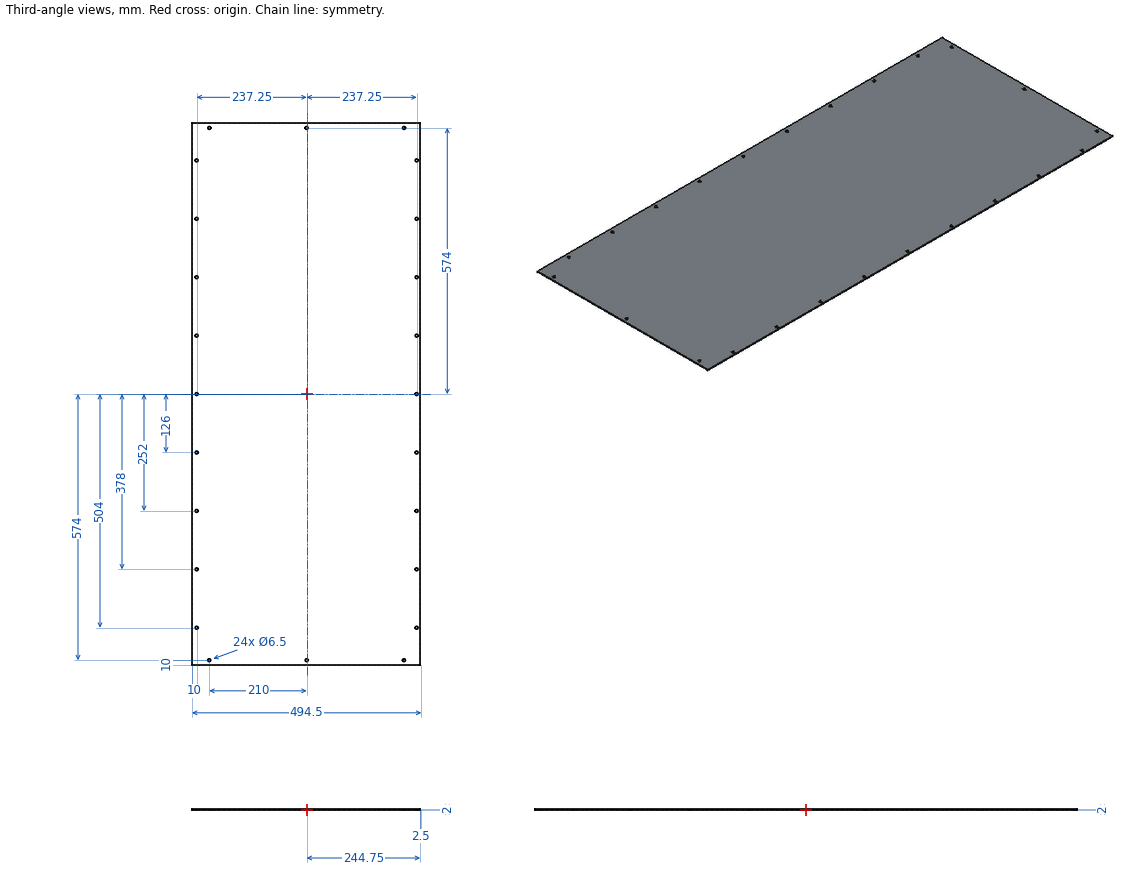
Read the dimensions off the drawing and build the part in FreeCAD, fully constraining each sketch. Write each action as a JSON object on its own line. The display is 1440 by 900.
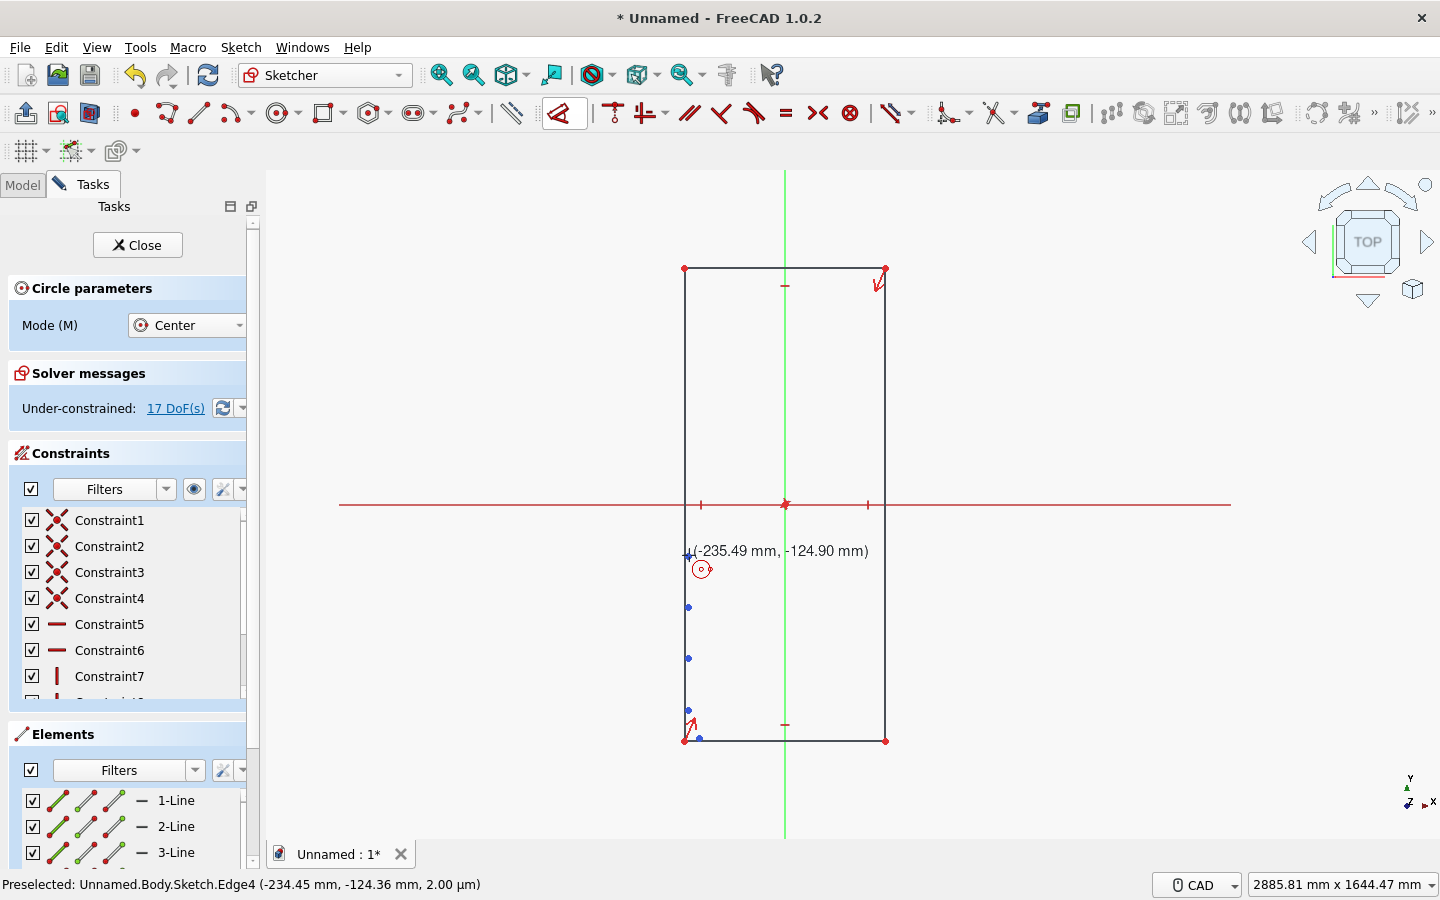
{"action": "scroll", "coordinate": [785, 738], "scroll_direction": "up", "scroll_amount": 15}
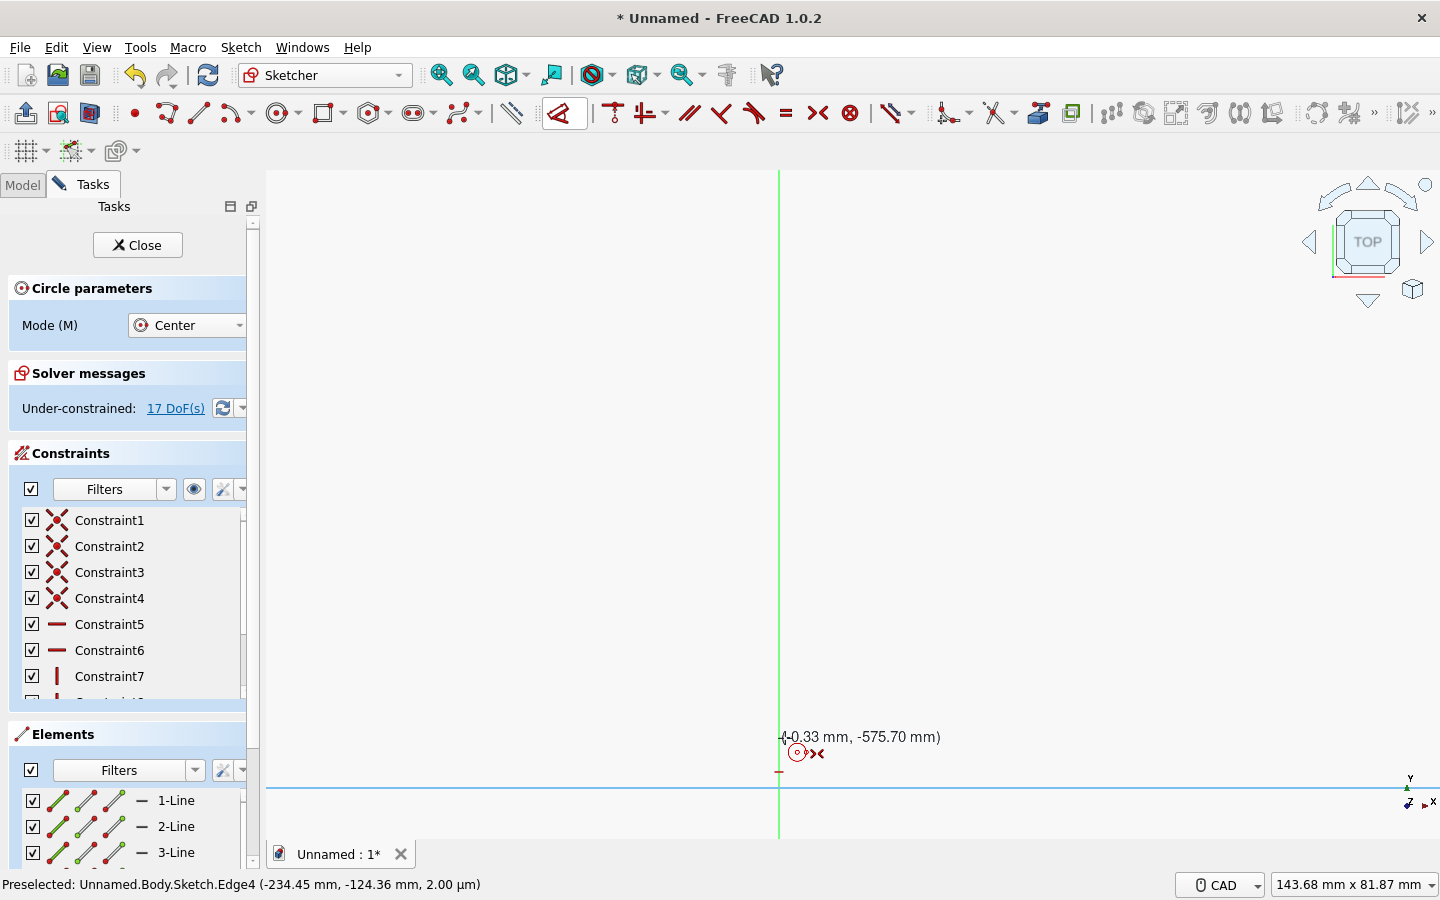
{"action": "scroll", "coordinate": [785, 739], "scroll_direction": "down", "scroll_amount": 15}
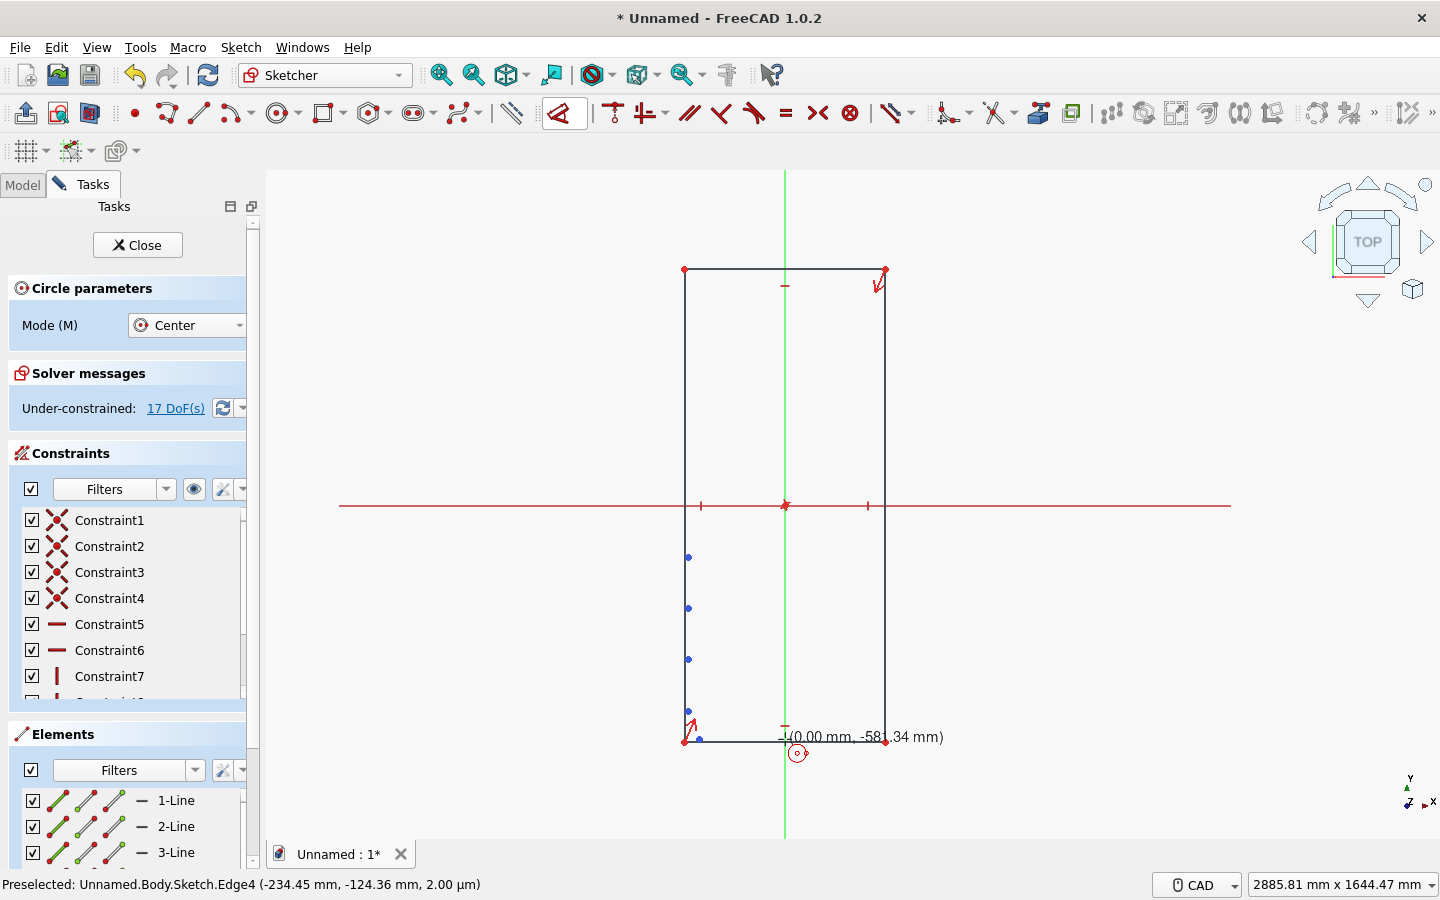
{"action": "scroll", "coordinate": [785, 739], "scroll_direction": "up", "scroll_amount": 7}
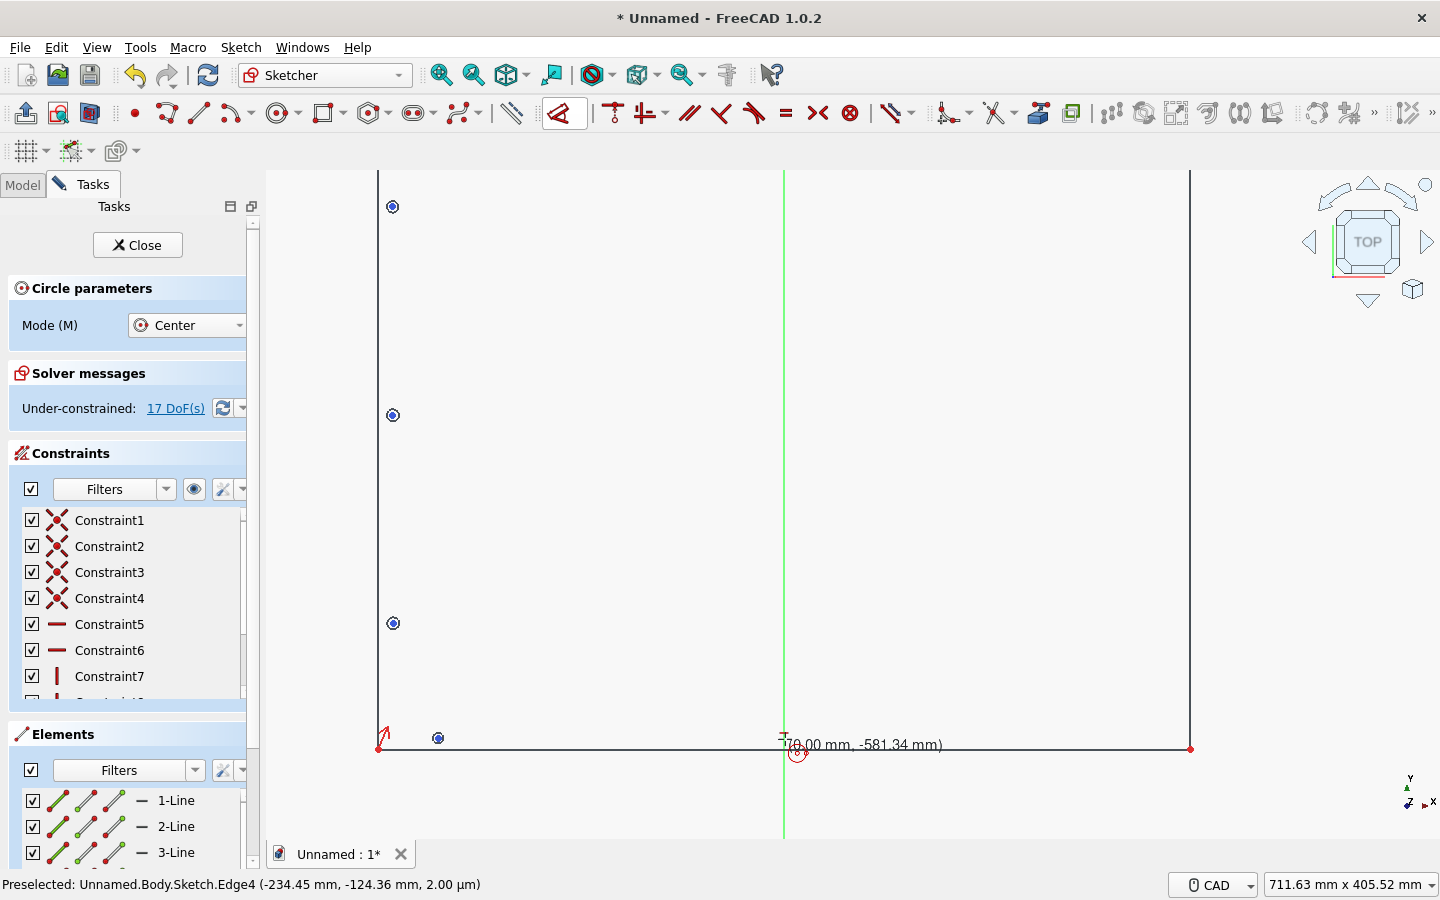
{"action": "left_click", "coordinate": [784, 737]}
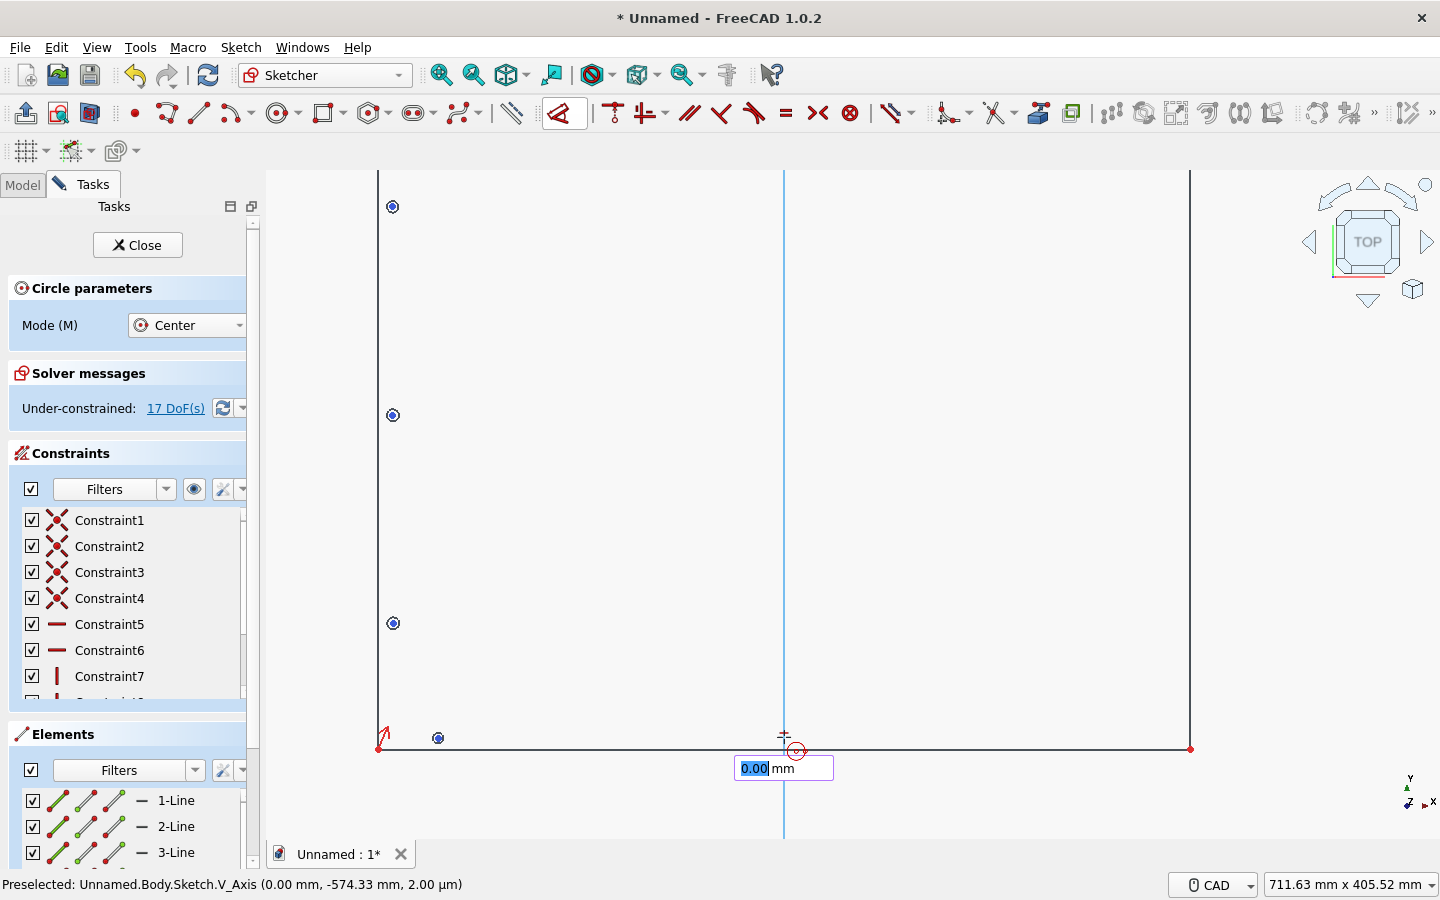
{"action": "scroll", "coordinate": [789, 736], "scroll_direction": "up", "scroll_amount": 6}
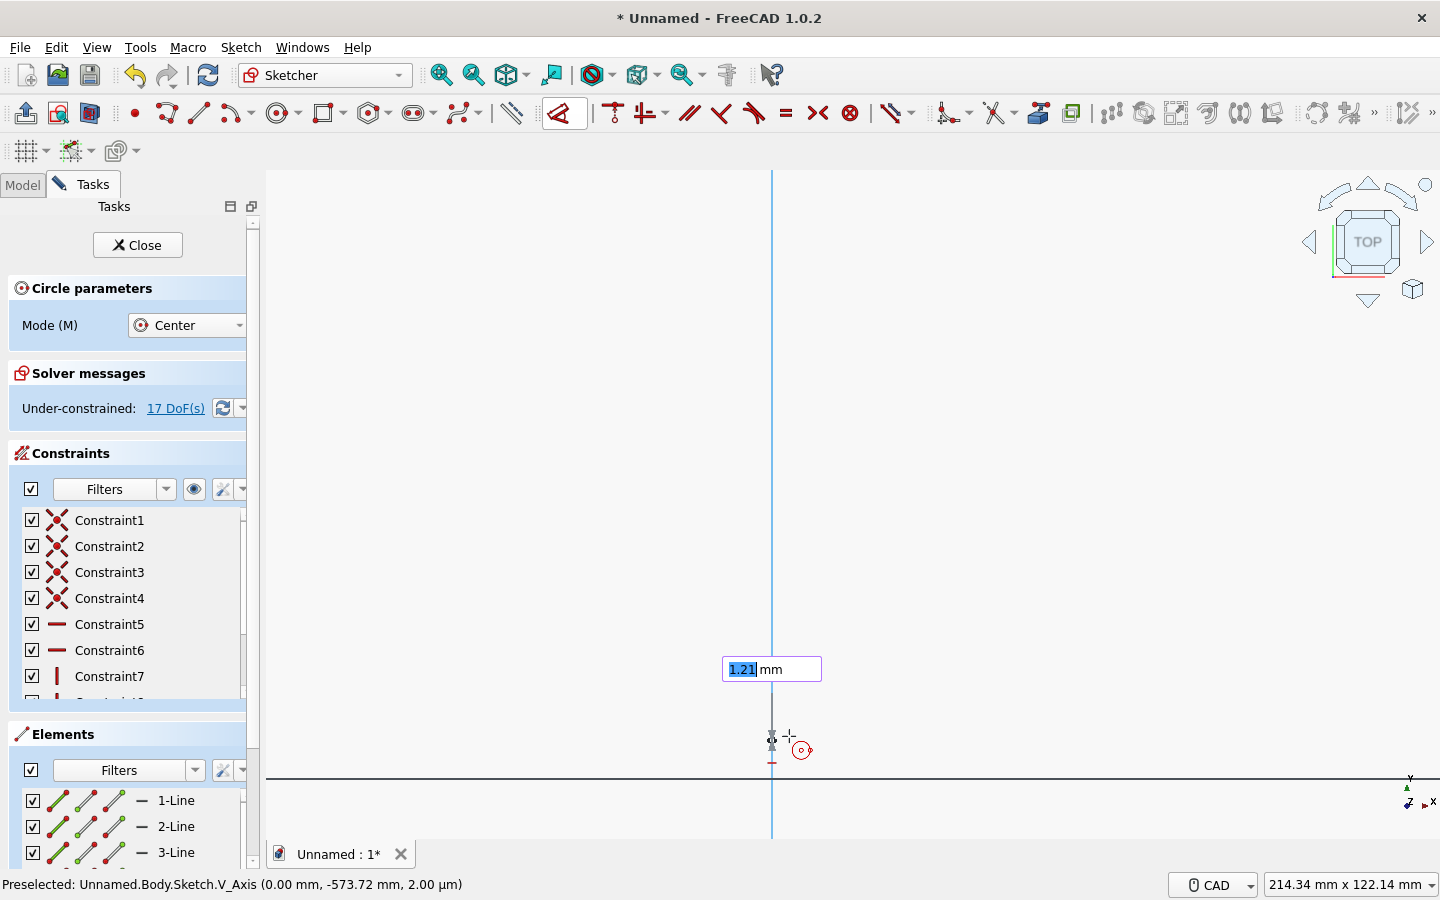
{"action": "left_click", "coordinate": [789, 733]}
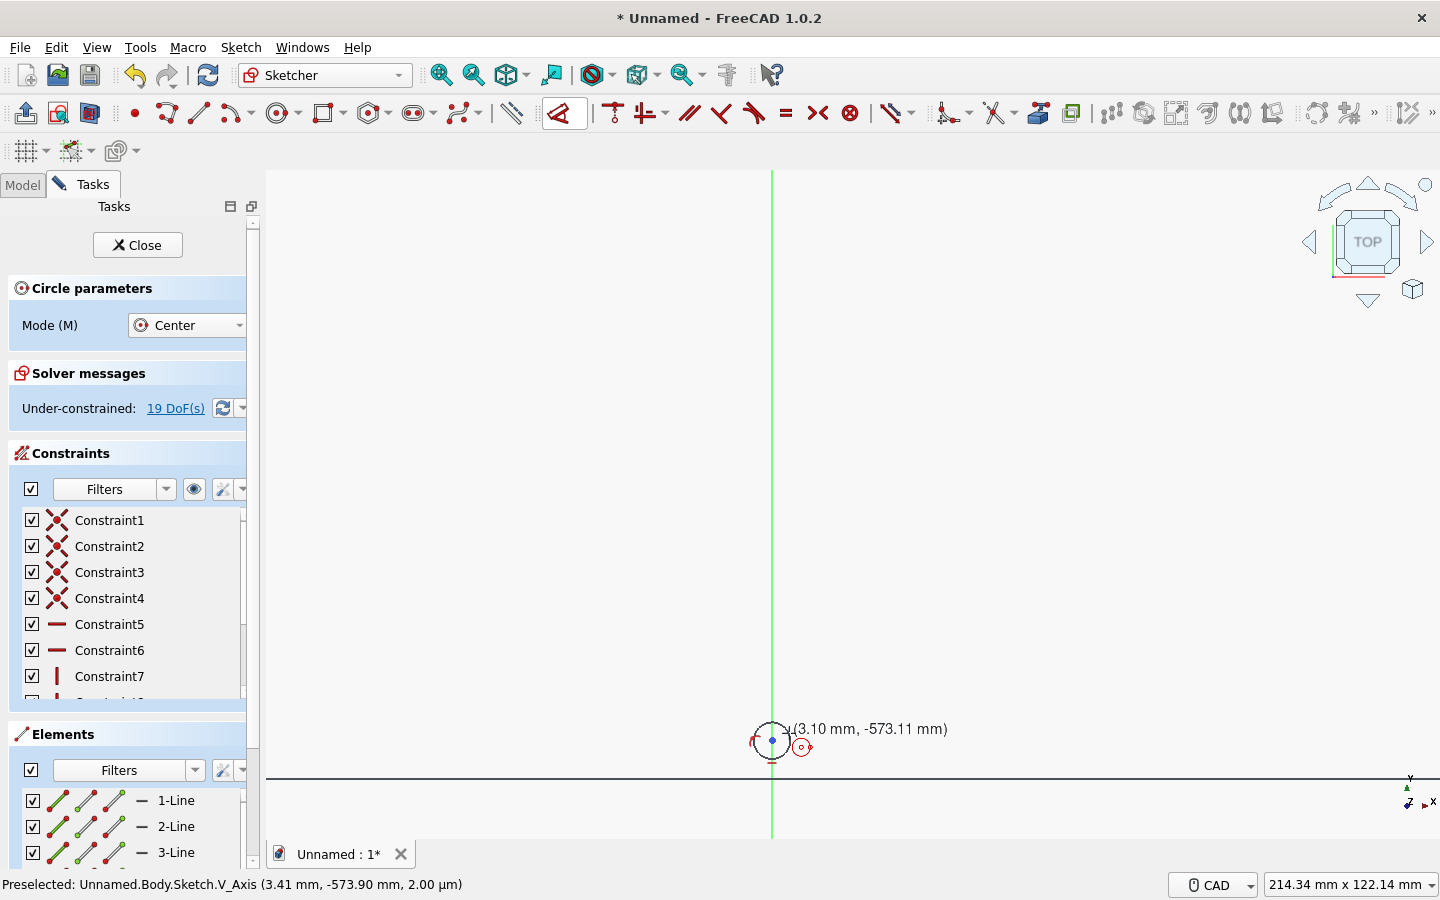
{"action": "scroll", "coordinate": [786, 738], "scroll_direction": "down", "scroll_amount": 13}